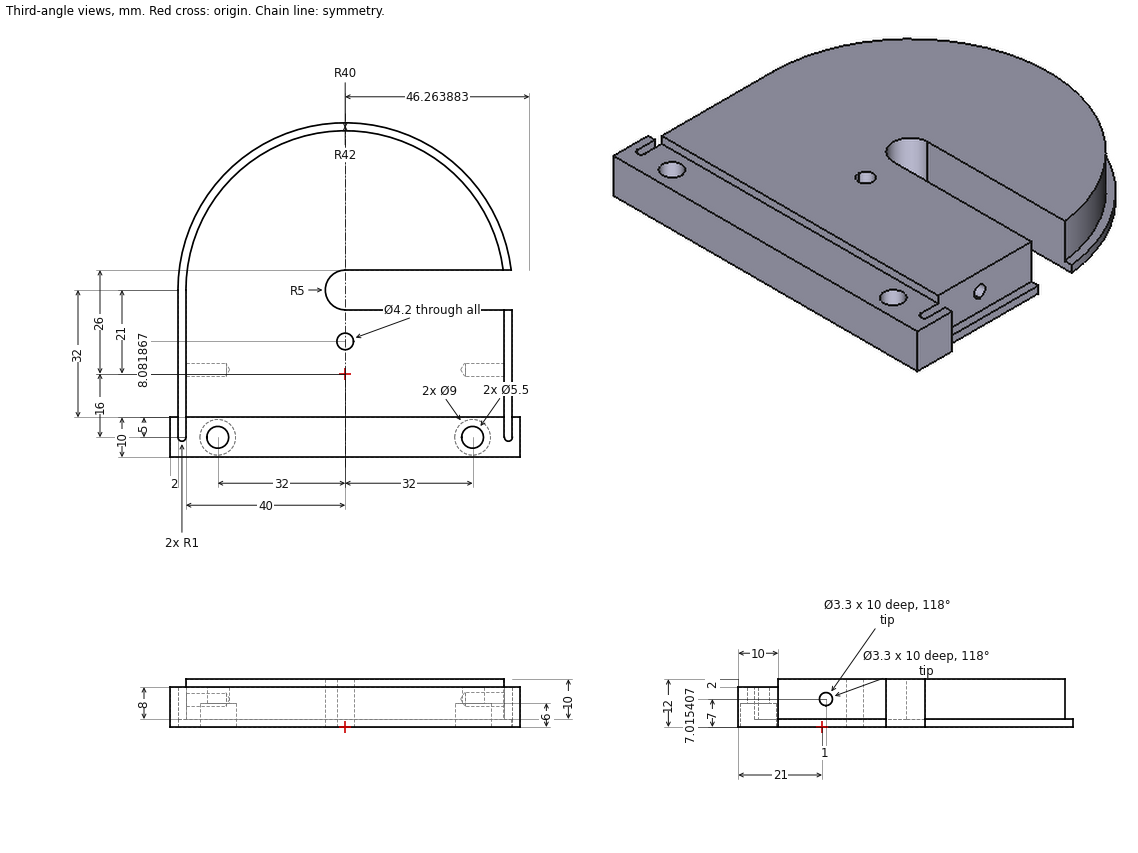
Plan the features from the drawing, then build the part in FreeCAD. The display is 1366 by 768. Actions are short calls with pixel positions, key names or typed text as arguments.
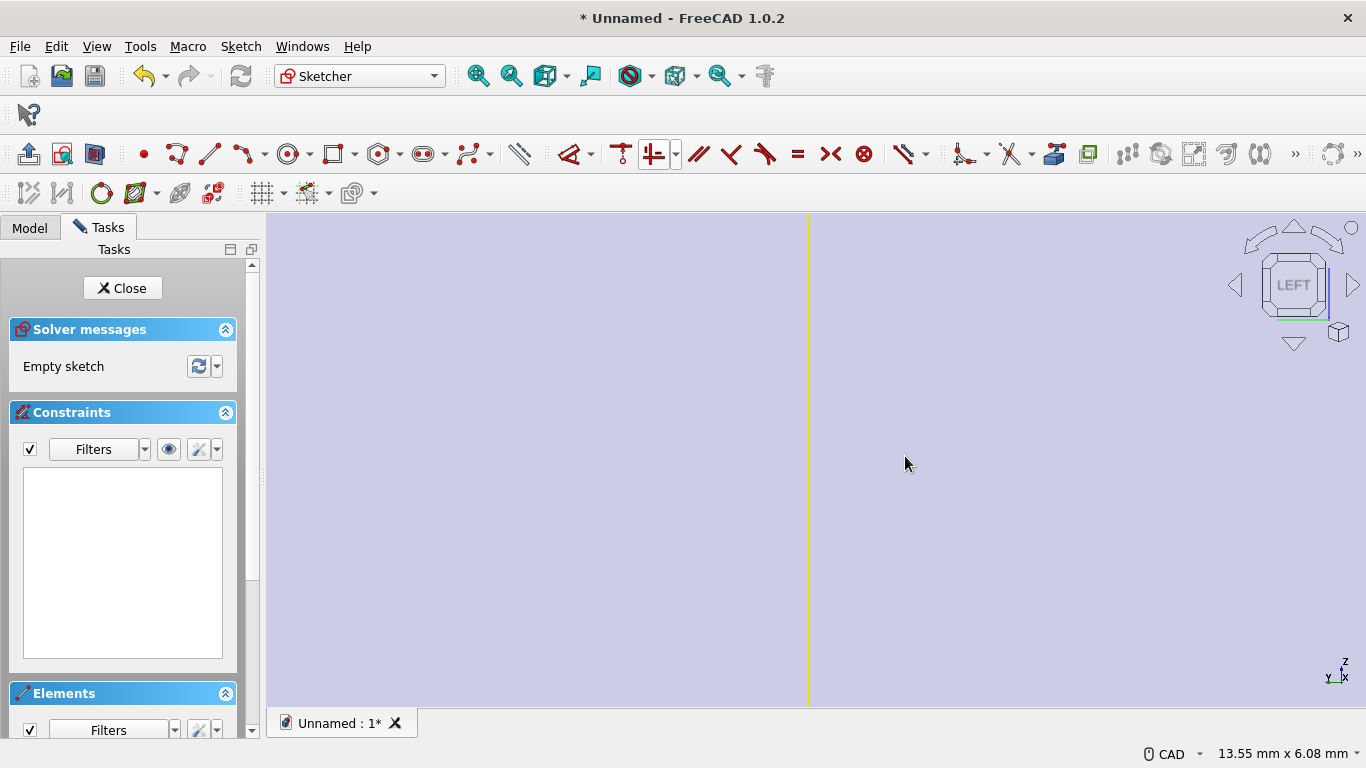
click(288, 154)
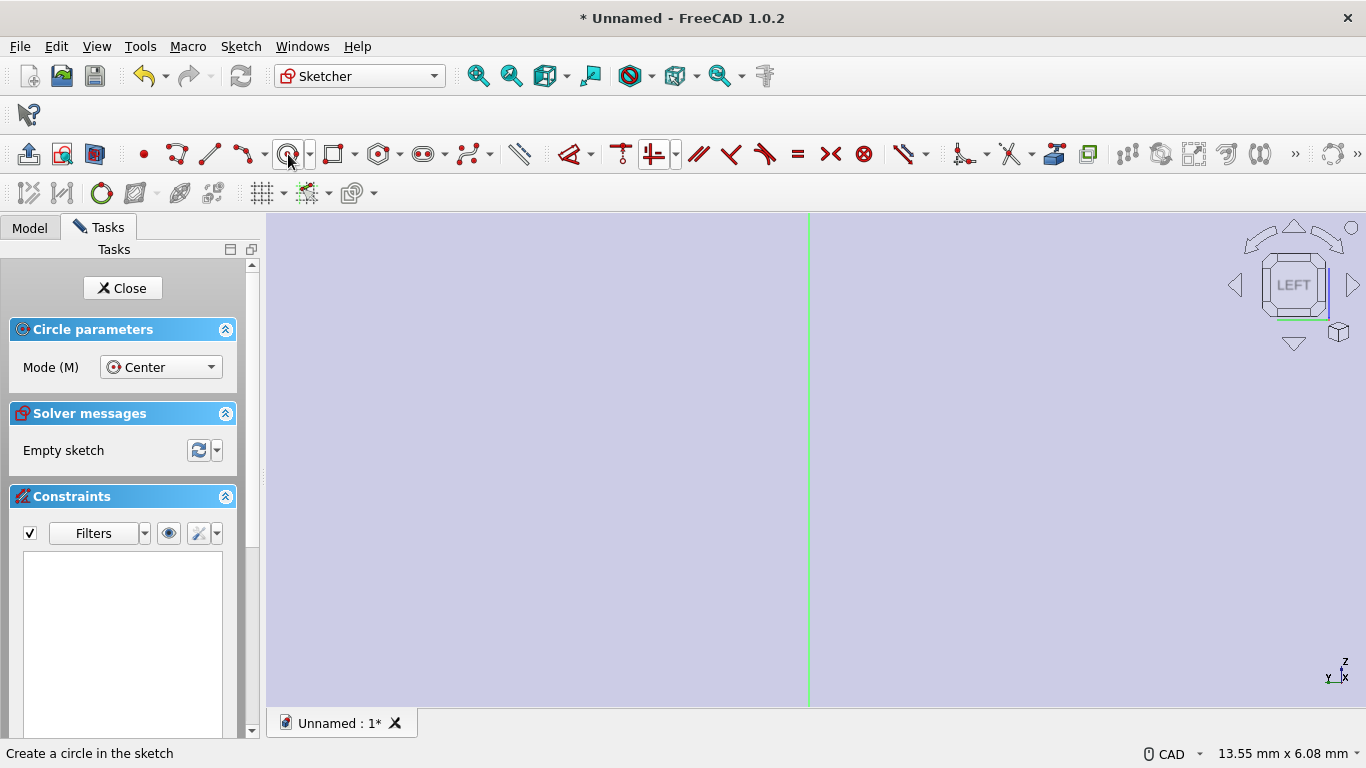
click(728, 446)
click(633, 351)
key(Escape)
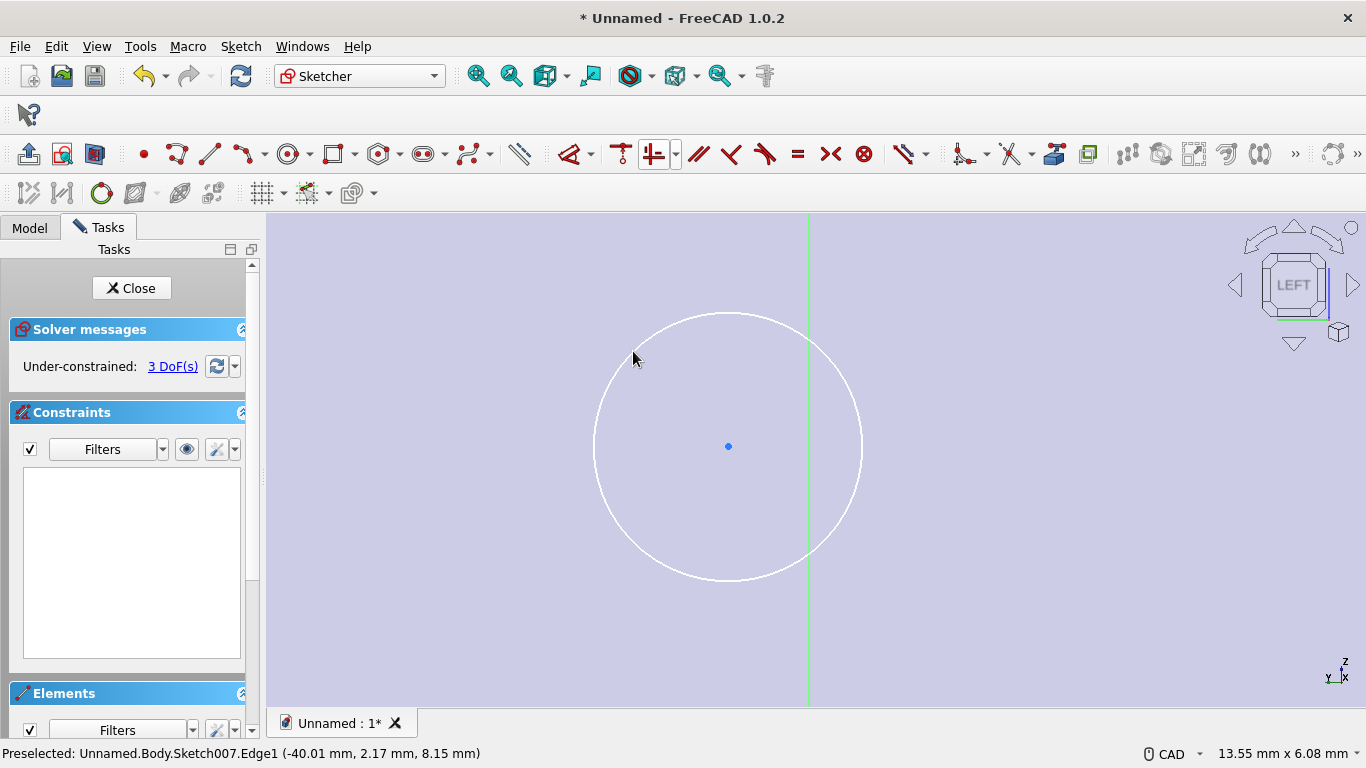
click(568, 154)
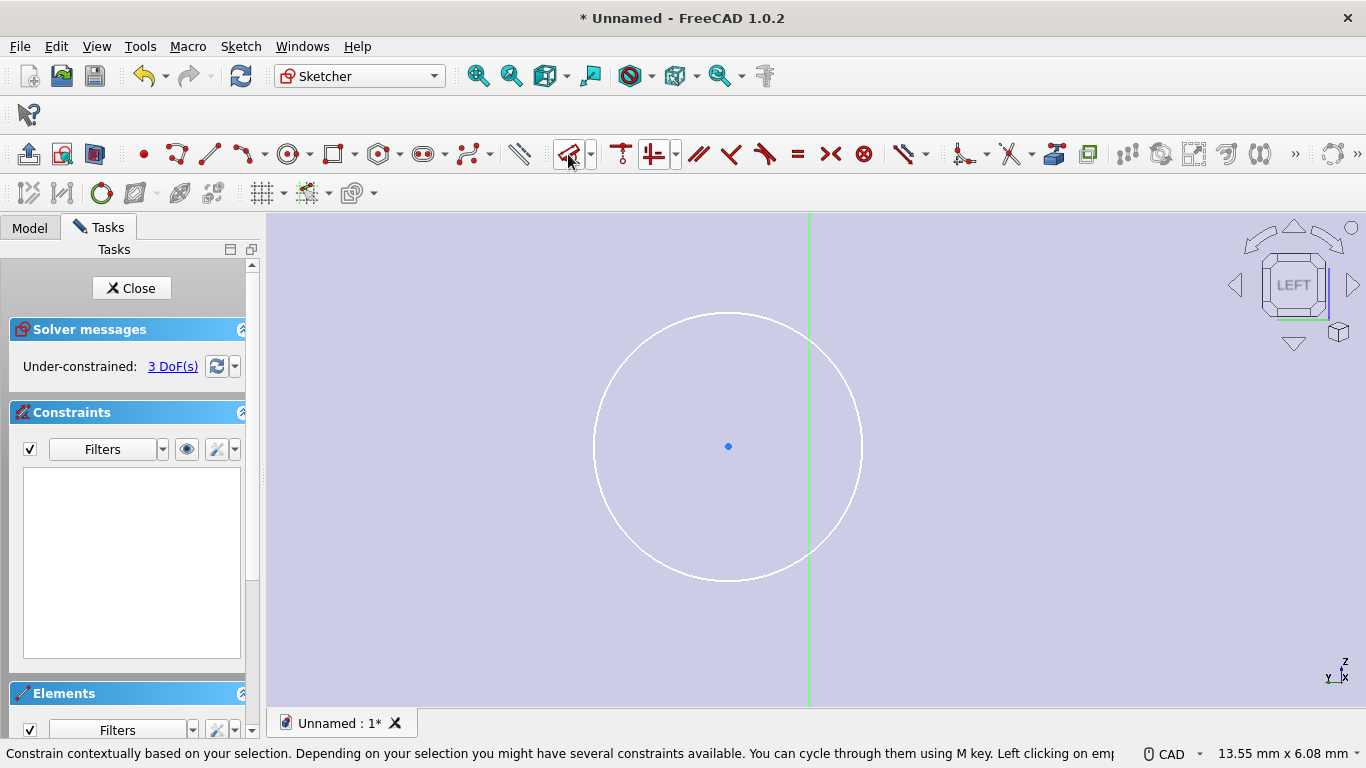
click(823, 352)
click(846, 329)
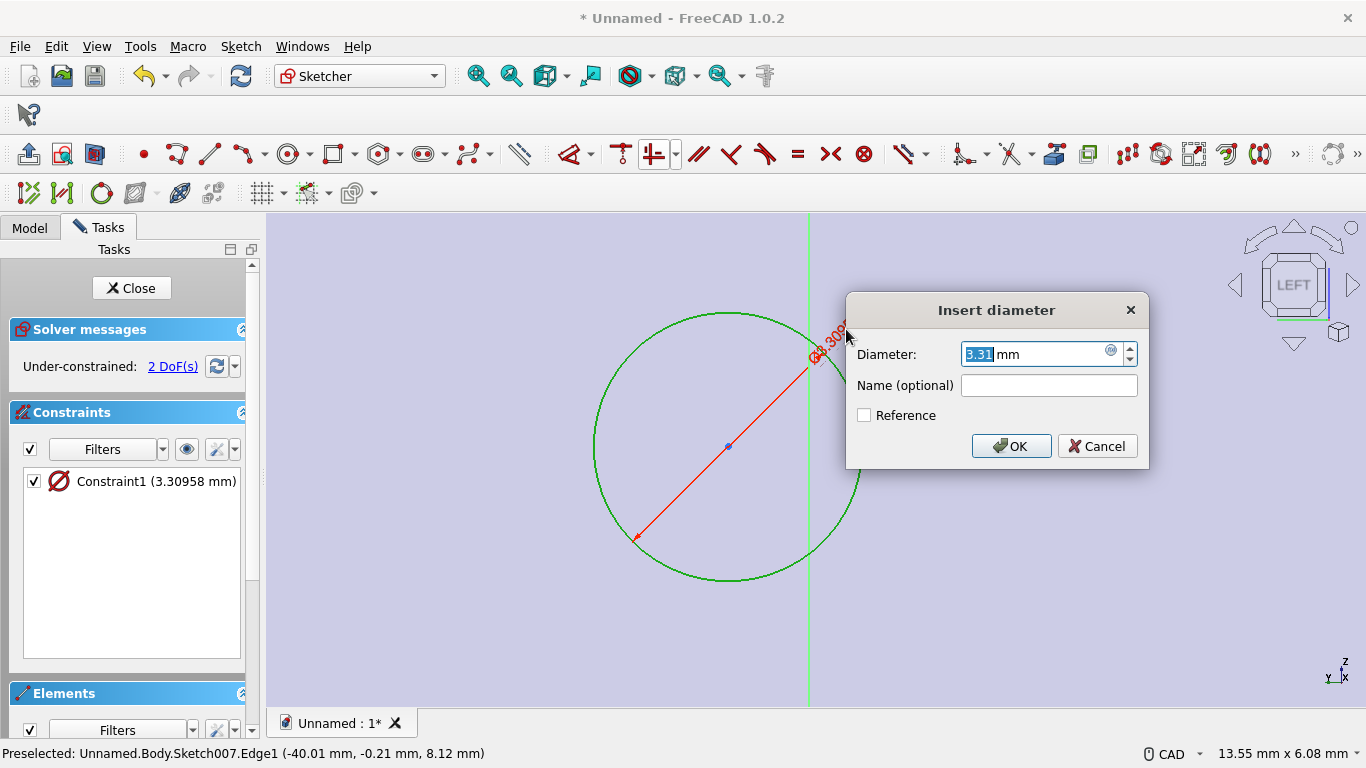
text(3.3)
key(Return)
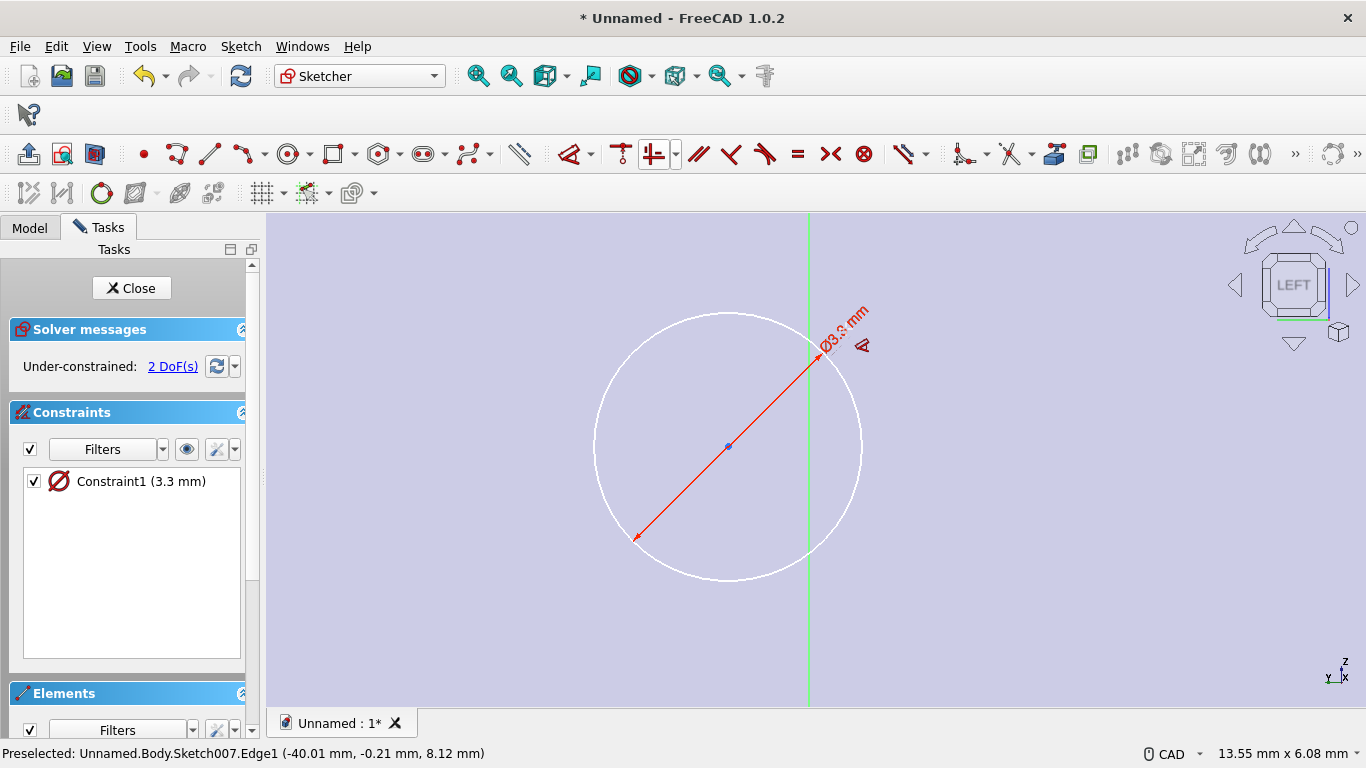
click(728, 447)
click(769, 413)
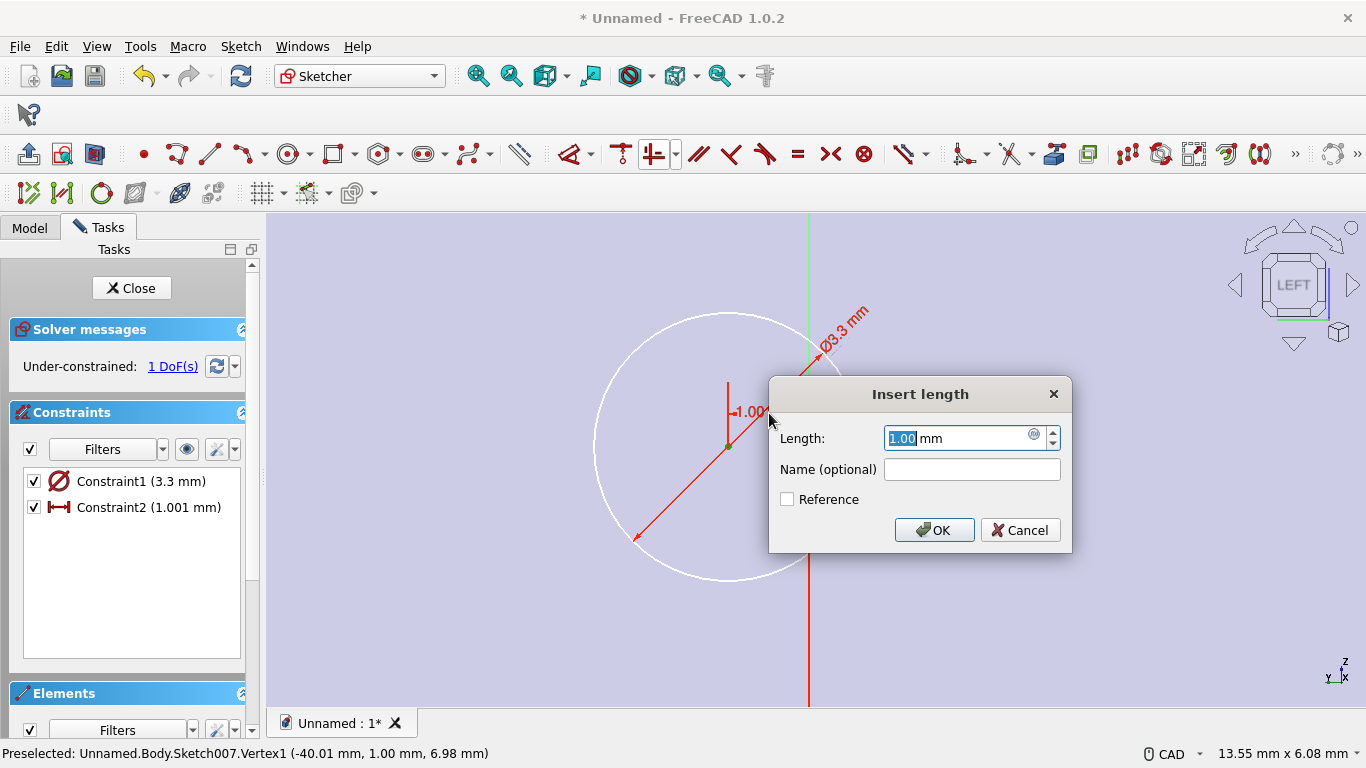
text(1)
key(Return)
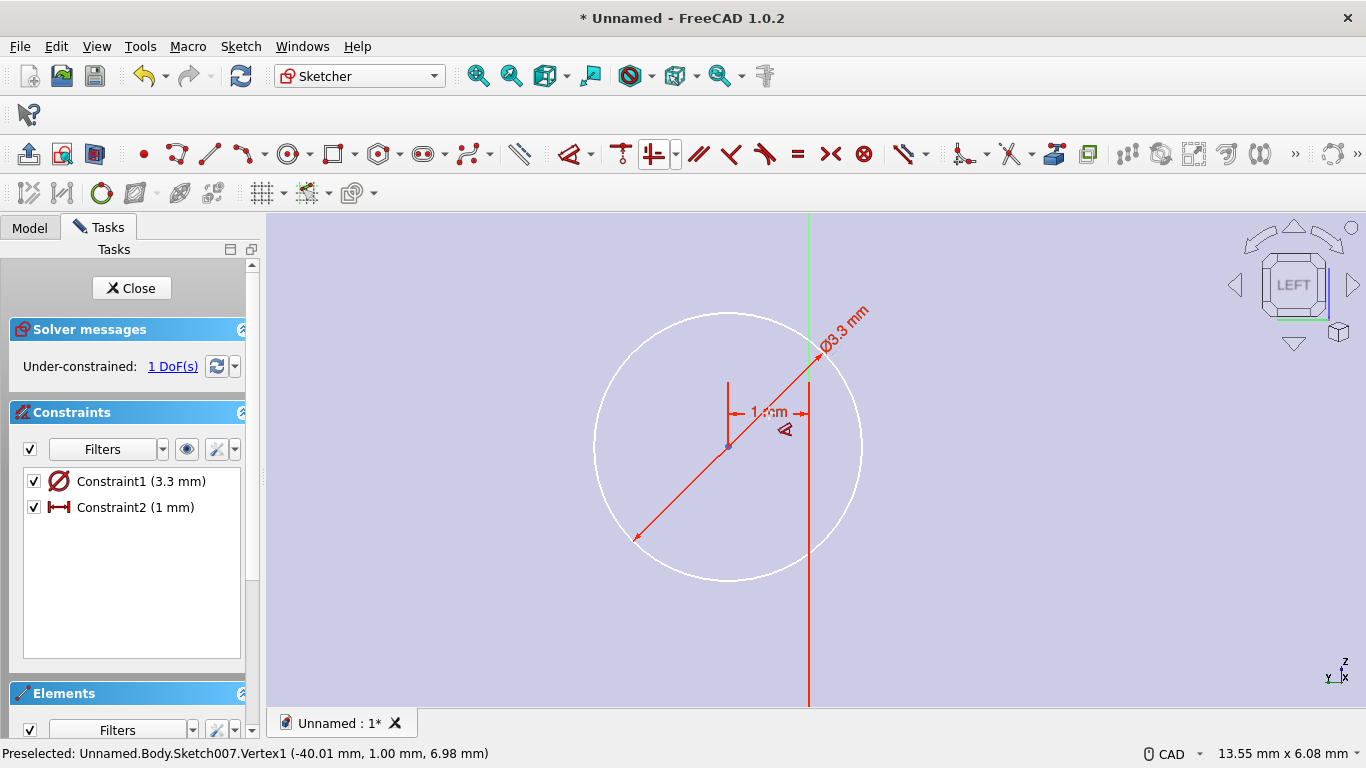
click(728, 447)
click(843, 563)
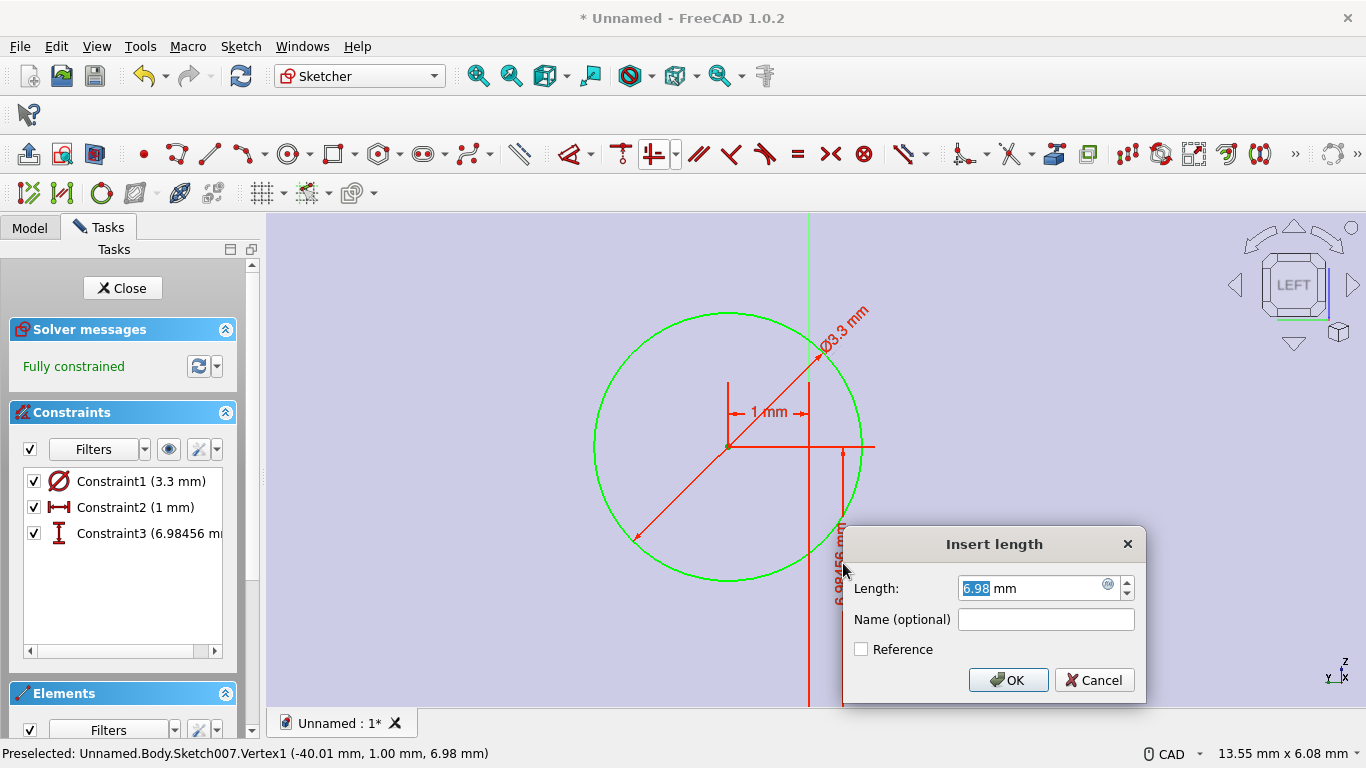
text(7)
key(Return)
key(Escape)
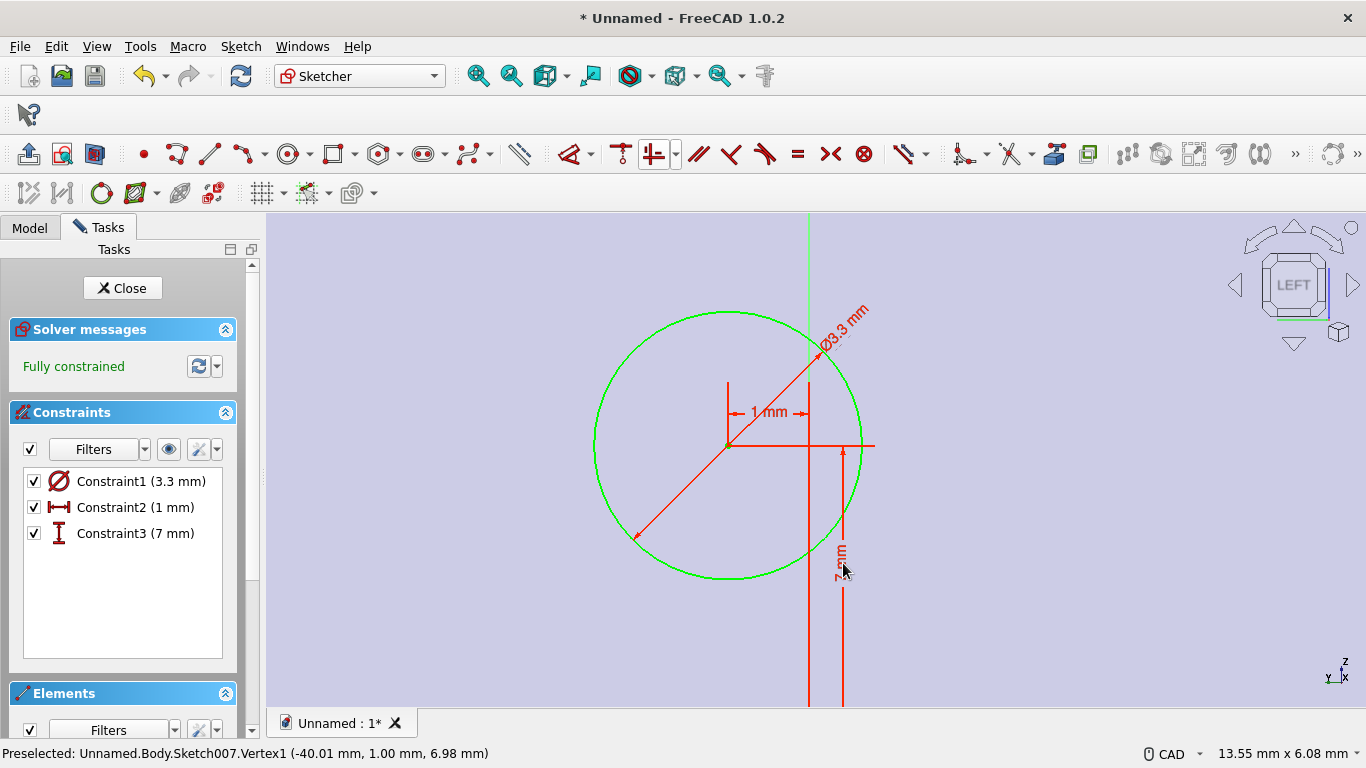
click(123, 288)